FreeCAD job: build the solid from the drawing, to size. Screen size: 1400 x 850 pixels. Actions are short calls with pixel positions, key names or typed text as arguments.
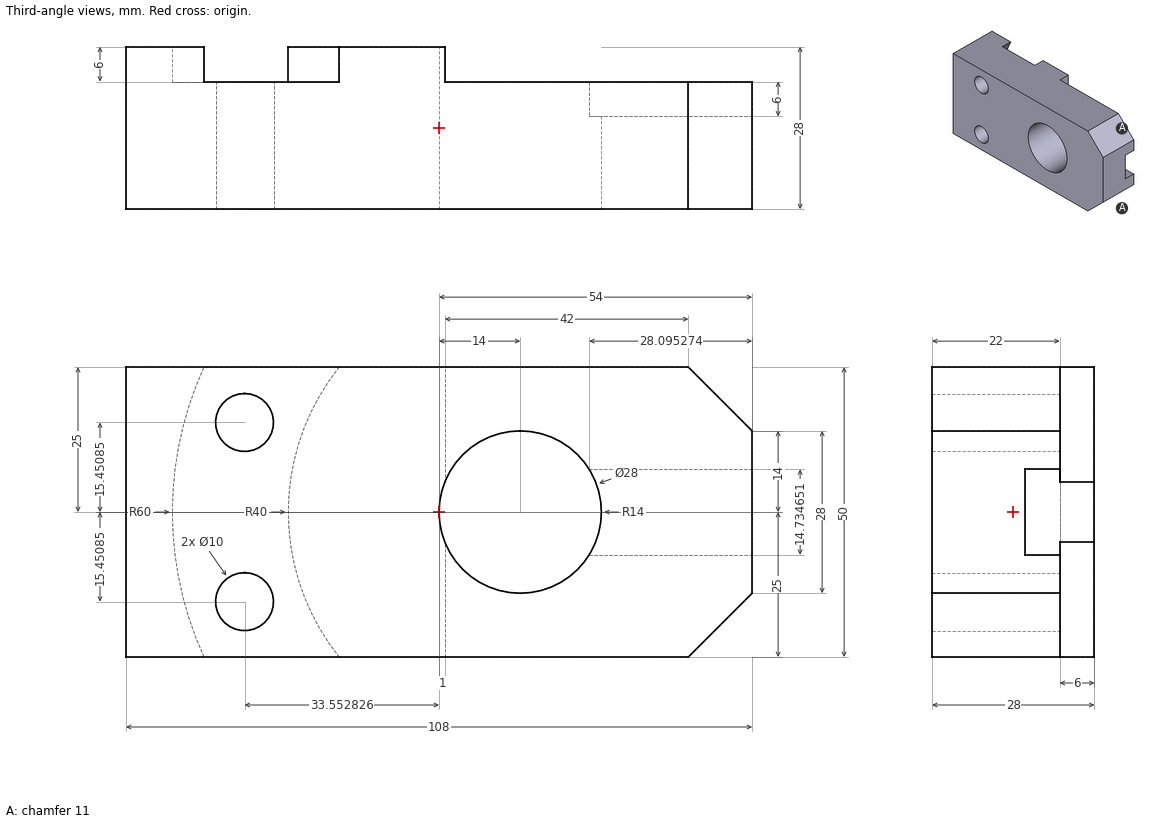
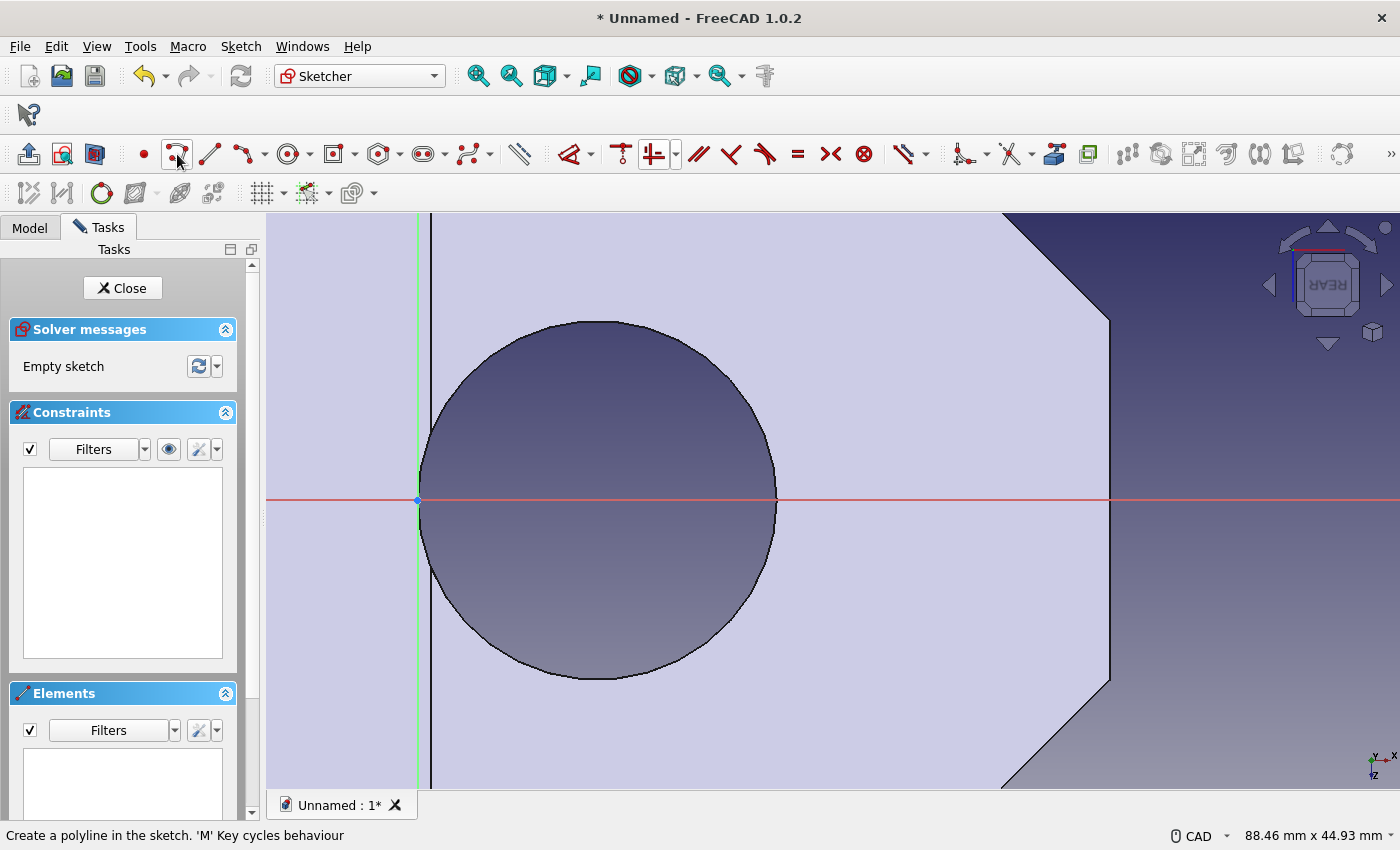
click(750, 595)
click(1110, 595)
click(1110, 406)
click(750, 406)
right_click(750, 406)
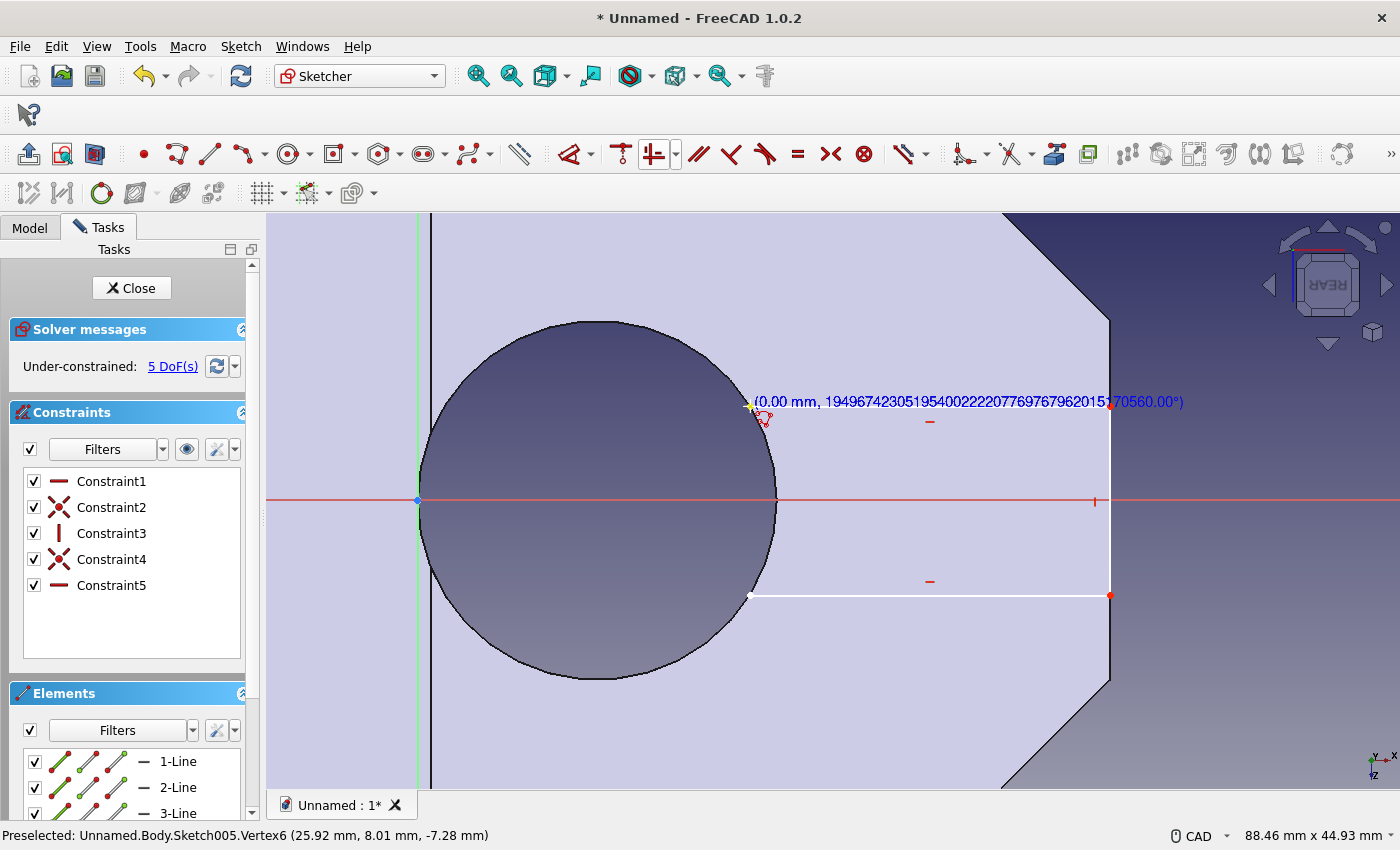
click(242, 154)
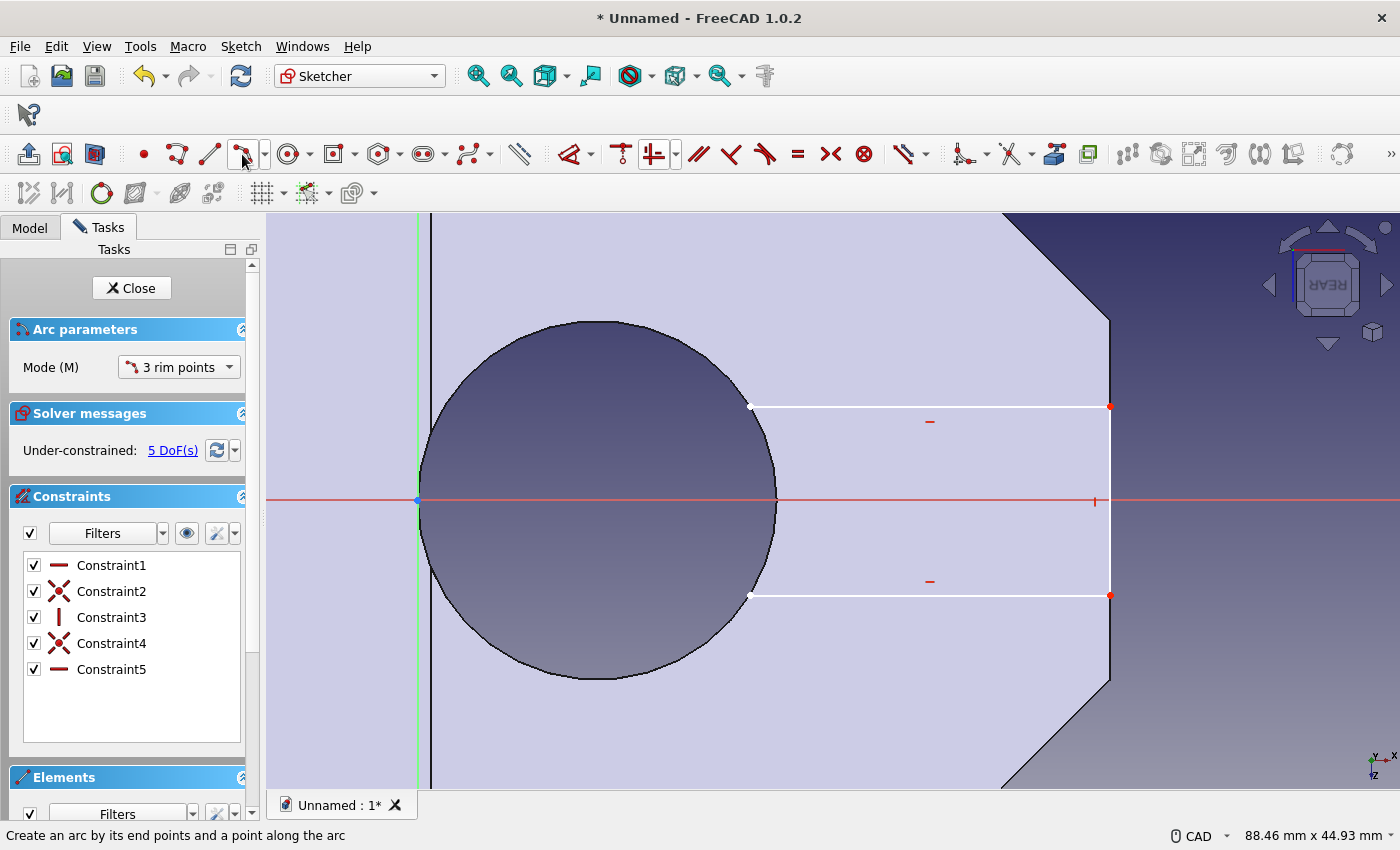
click(750, 407)
click(750, 596)
click(776, 520)
key(Escape)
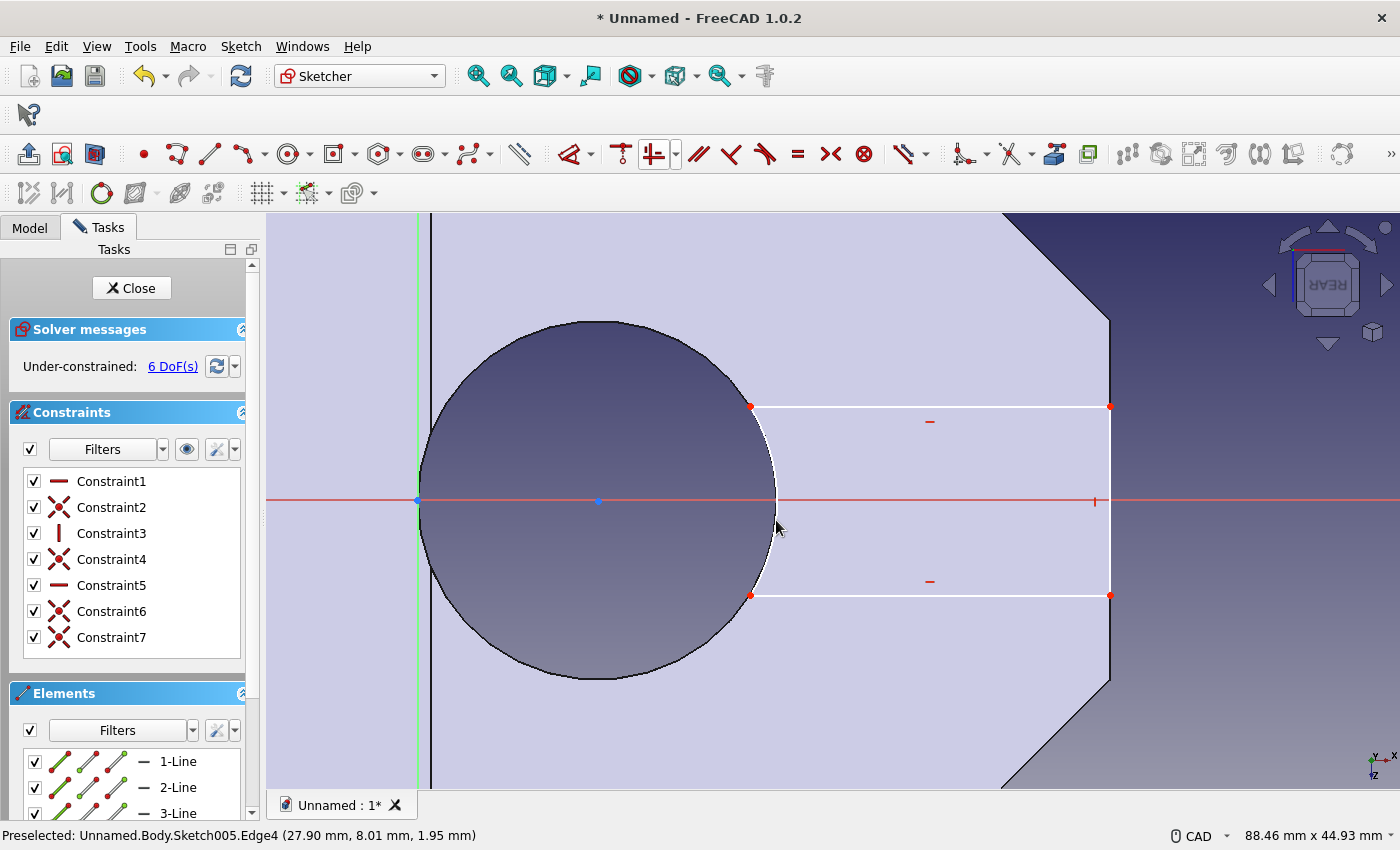
click(599, 501)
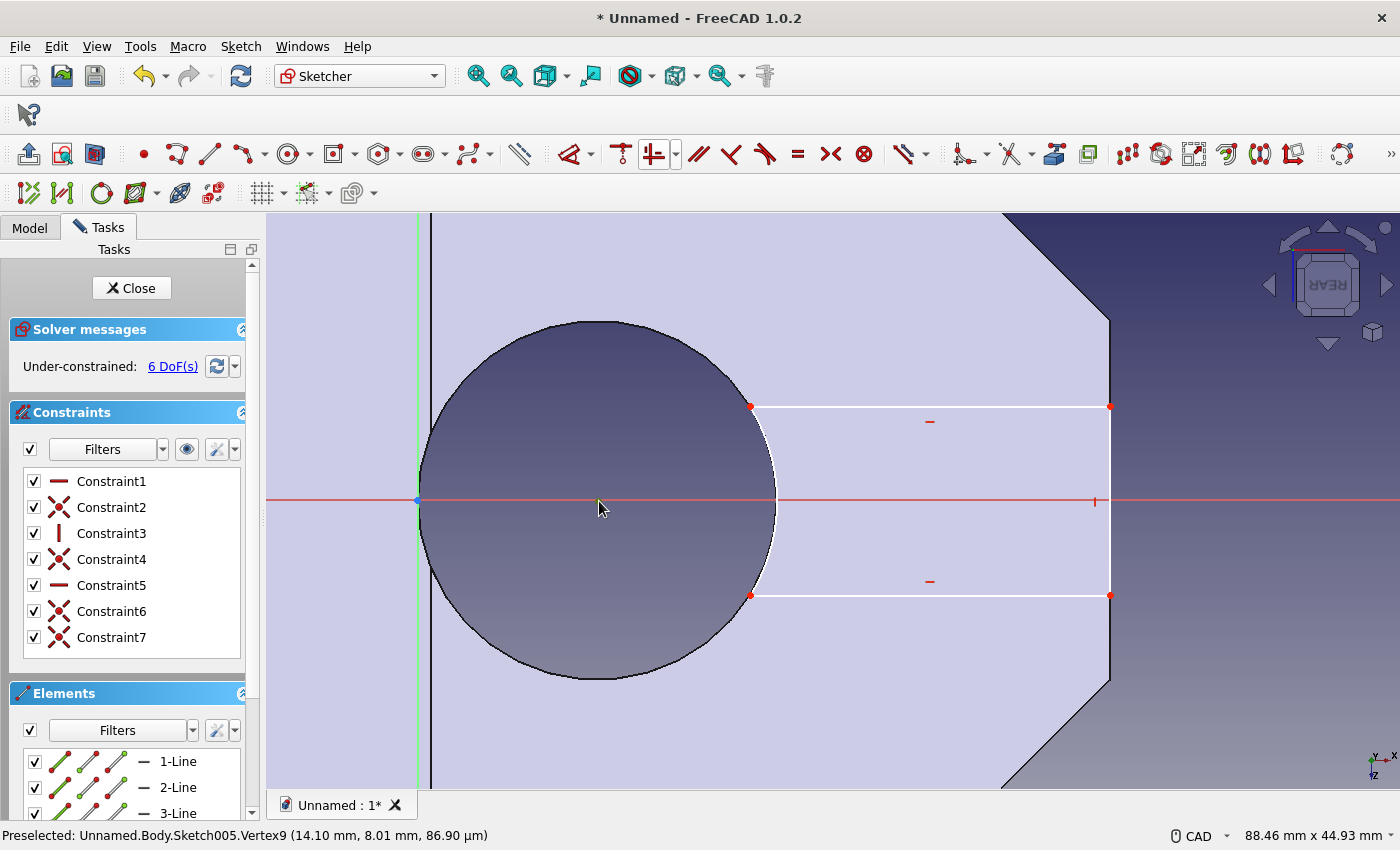
click(361, 500)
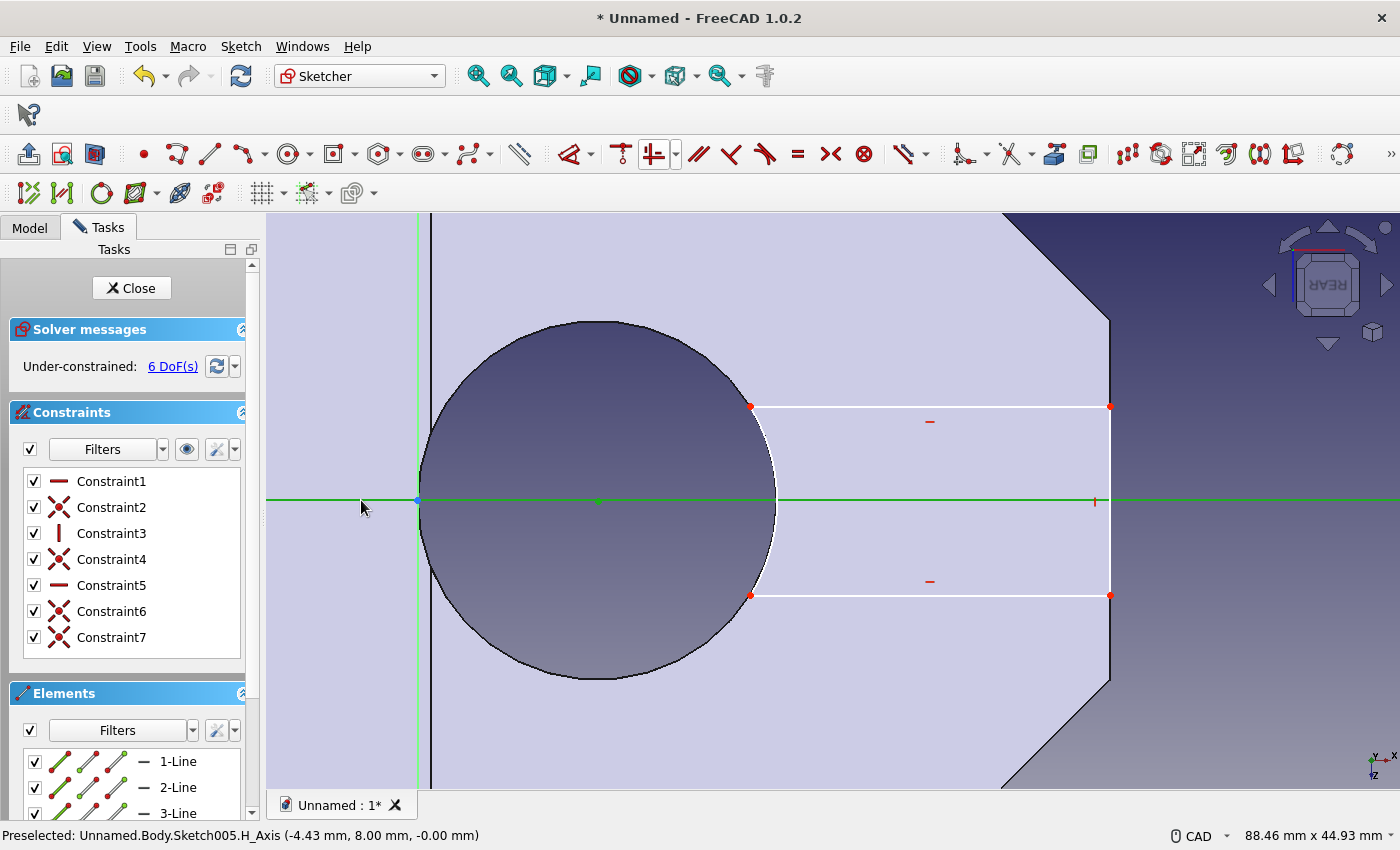
click(621, 154)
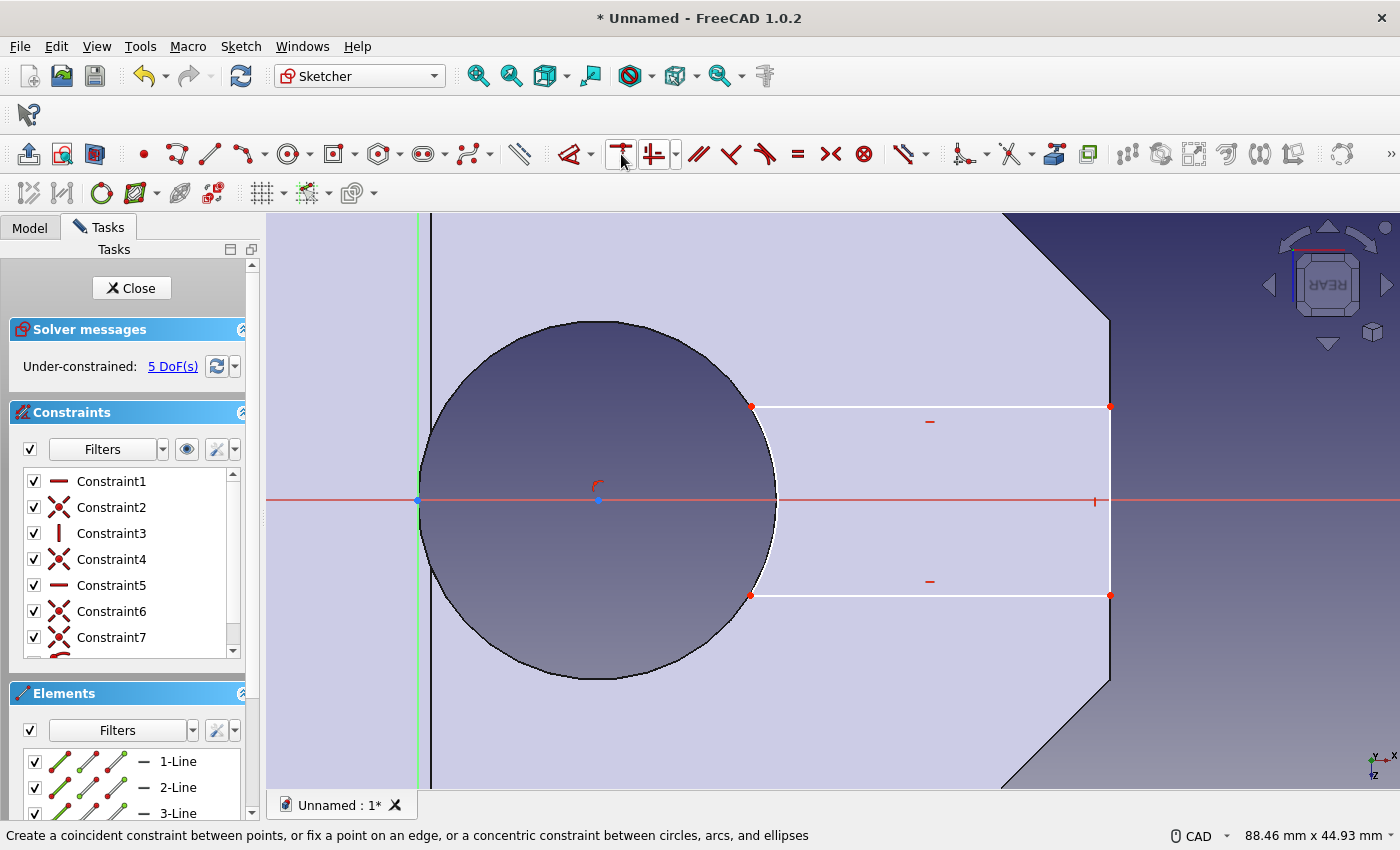
key(d)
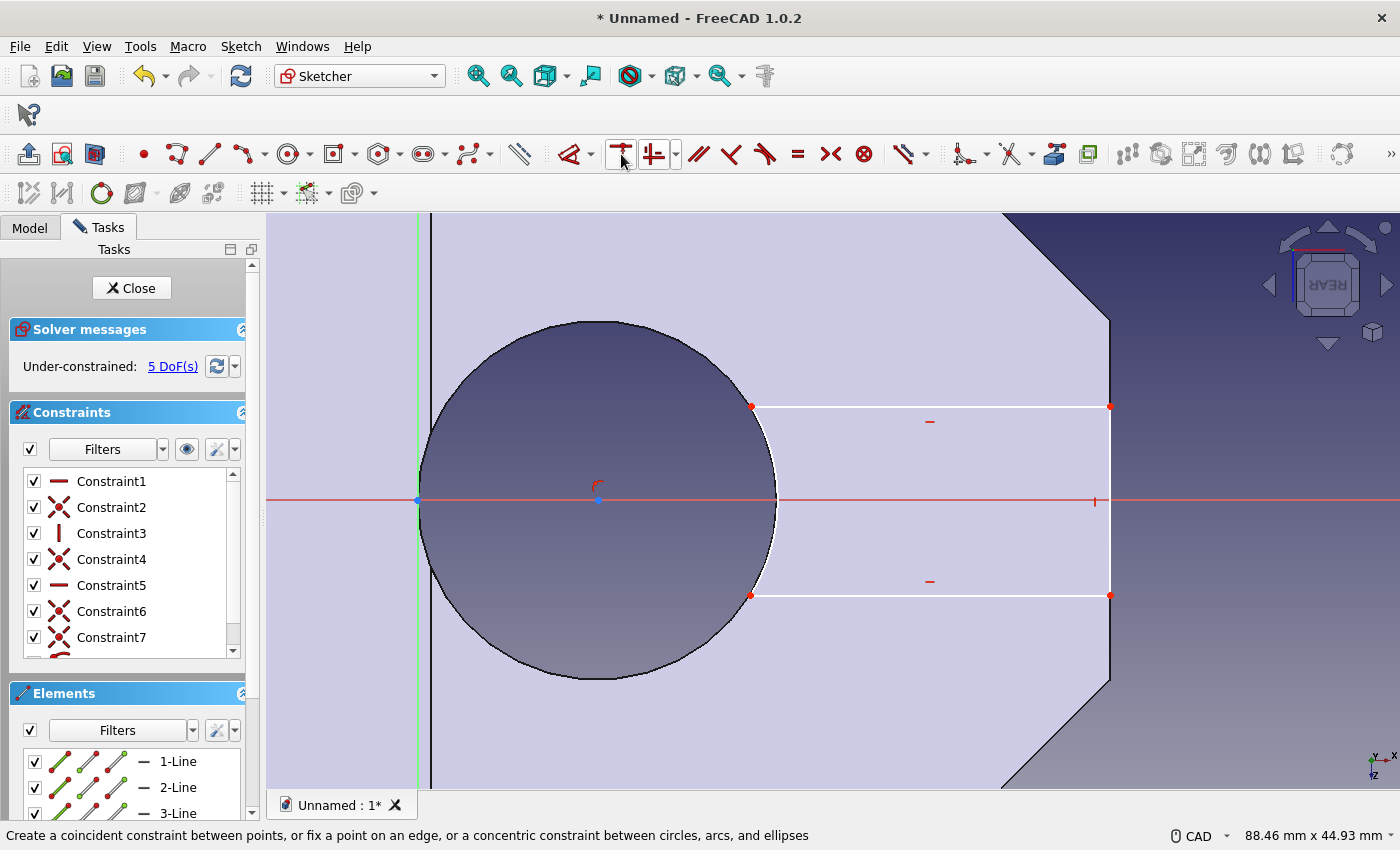
click(773, 541)
click(804, 548)